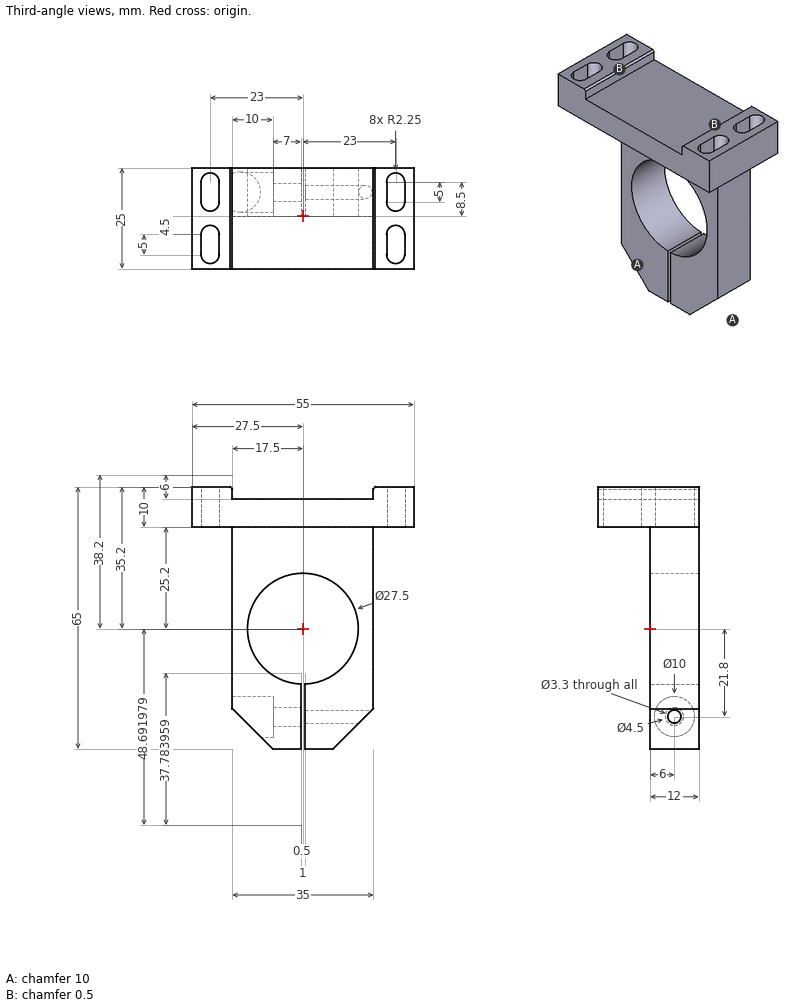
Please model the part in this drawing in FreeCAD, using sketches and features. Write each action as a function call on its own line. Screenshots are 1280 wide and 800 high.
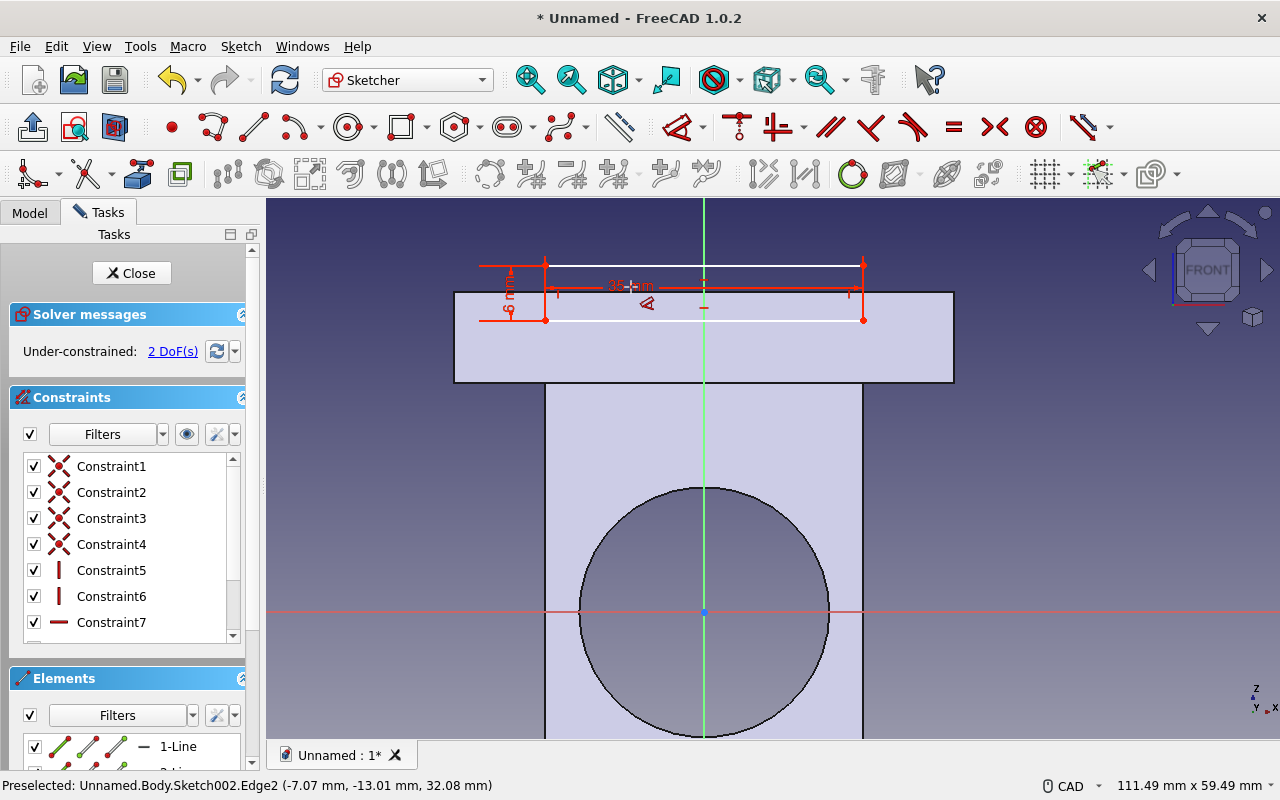
click(545, 266)
click(625, 646)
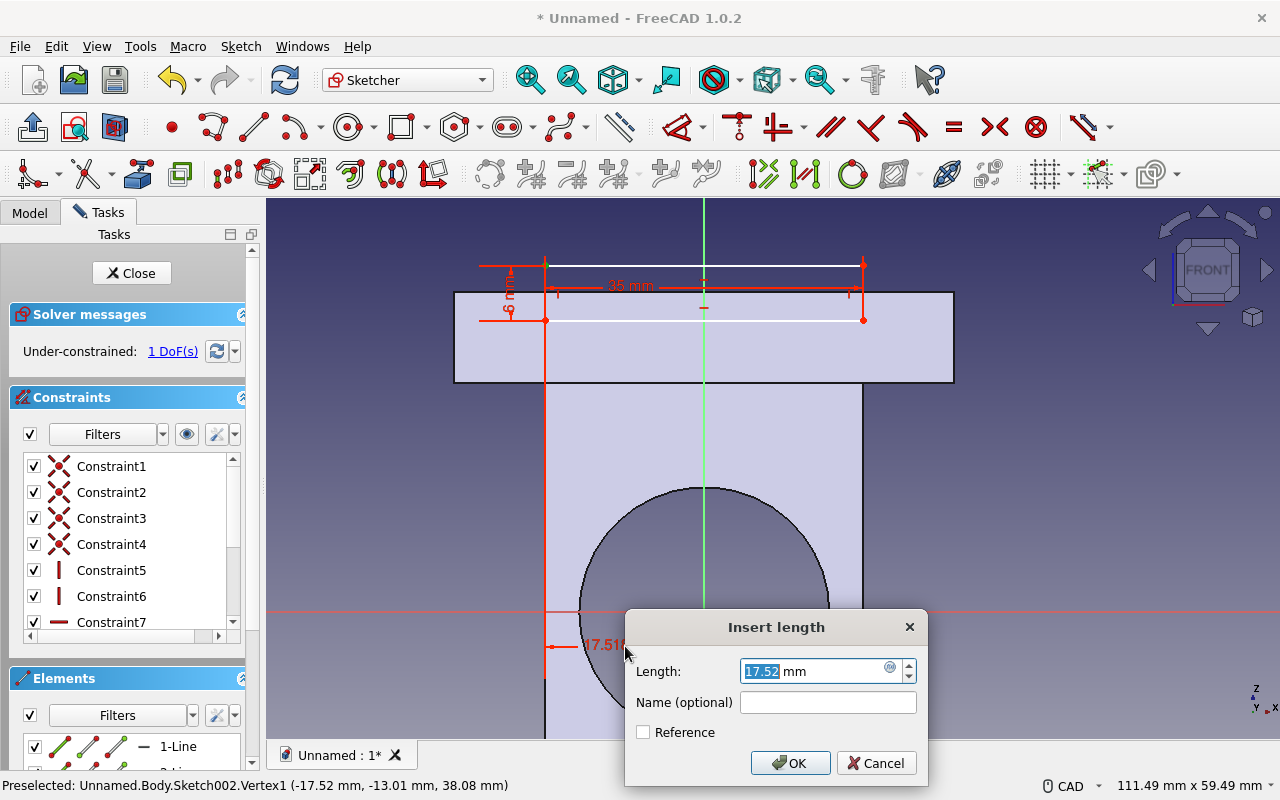
text(17.5)
key(Return)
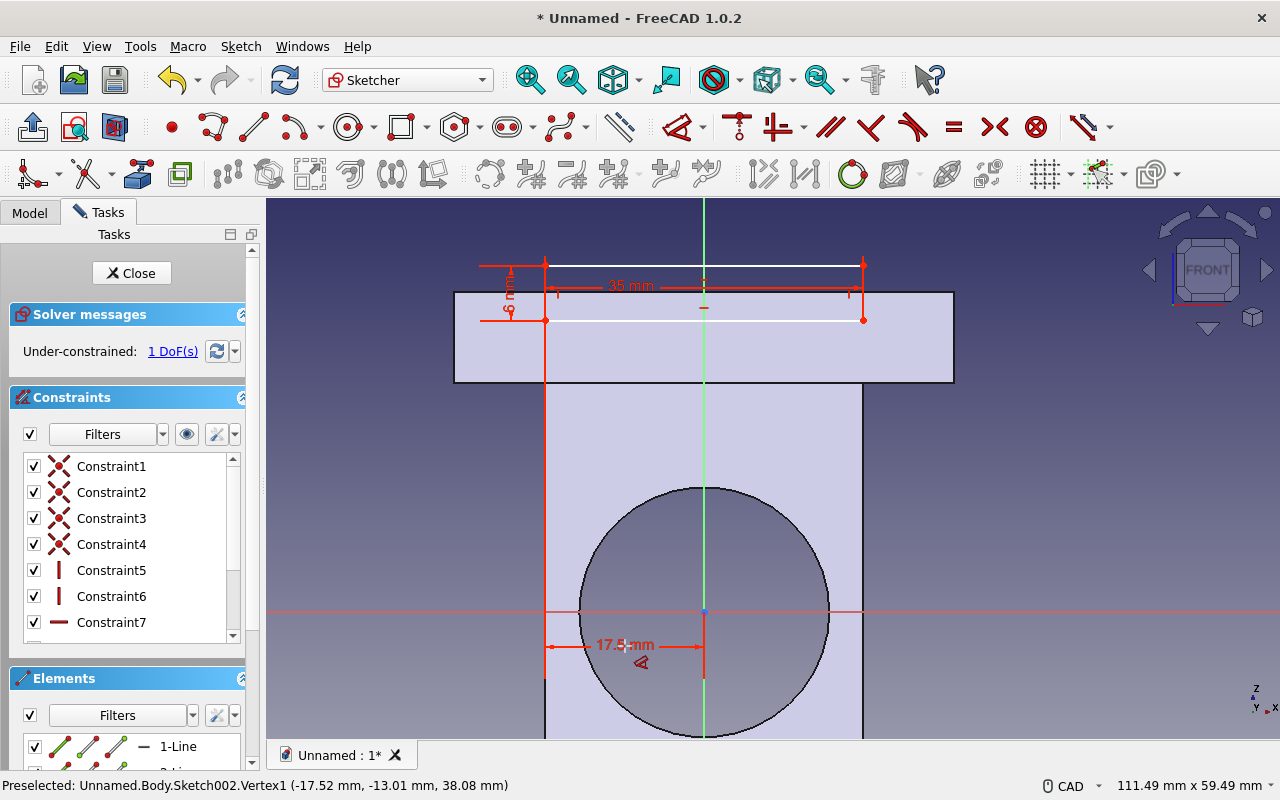
click(545, 266)
click(511, 439)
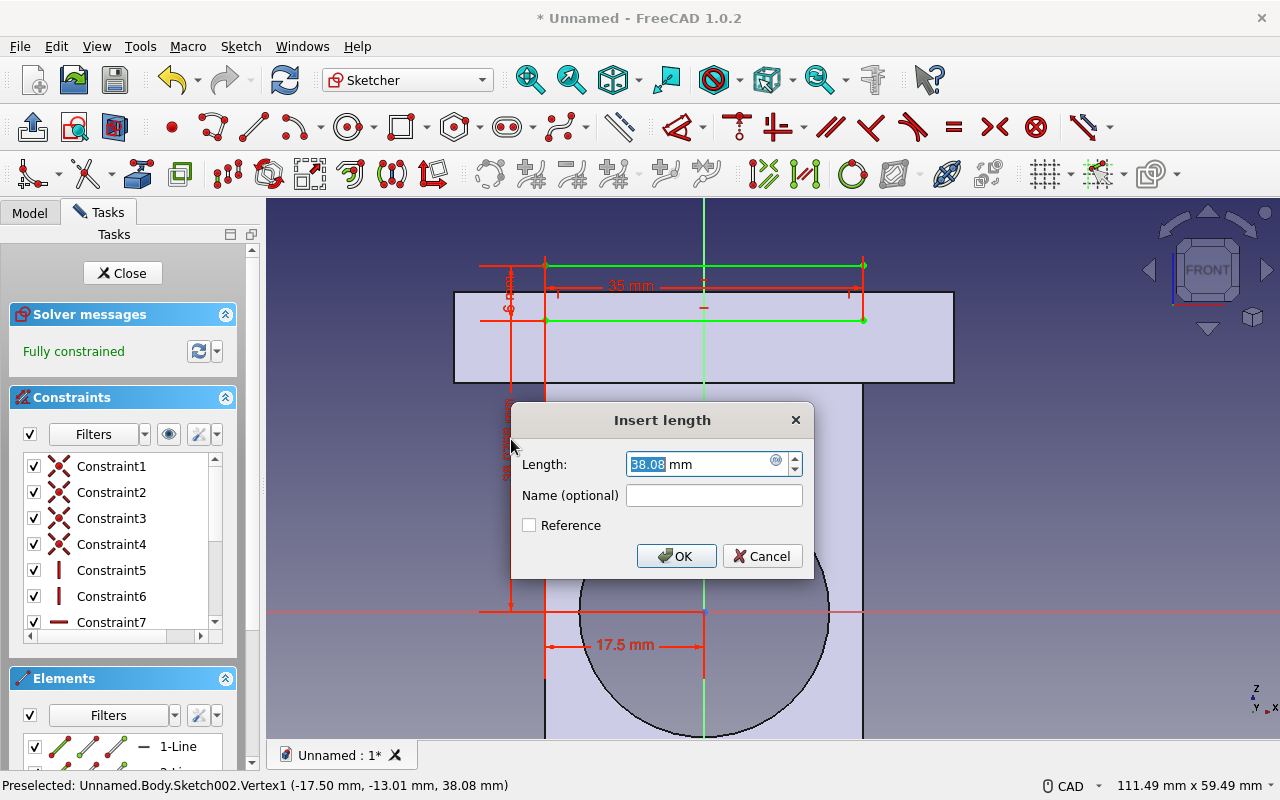
text(38.2)
key(Return)
key(Escape)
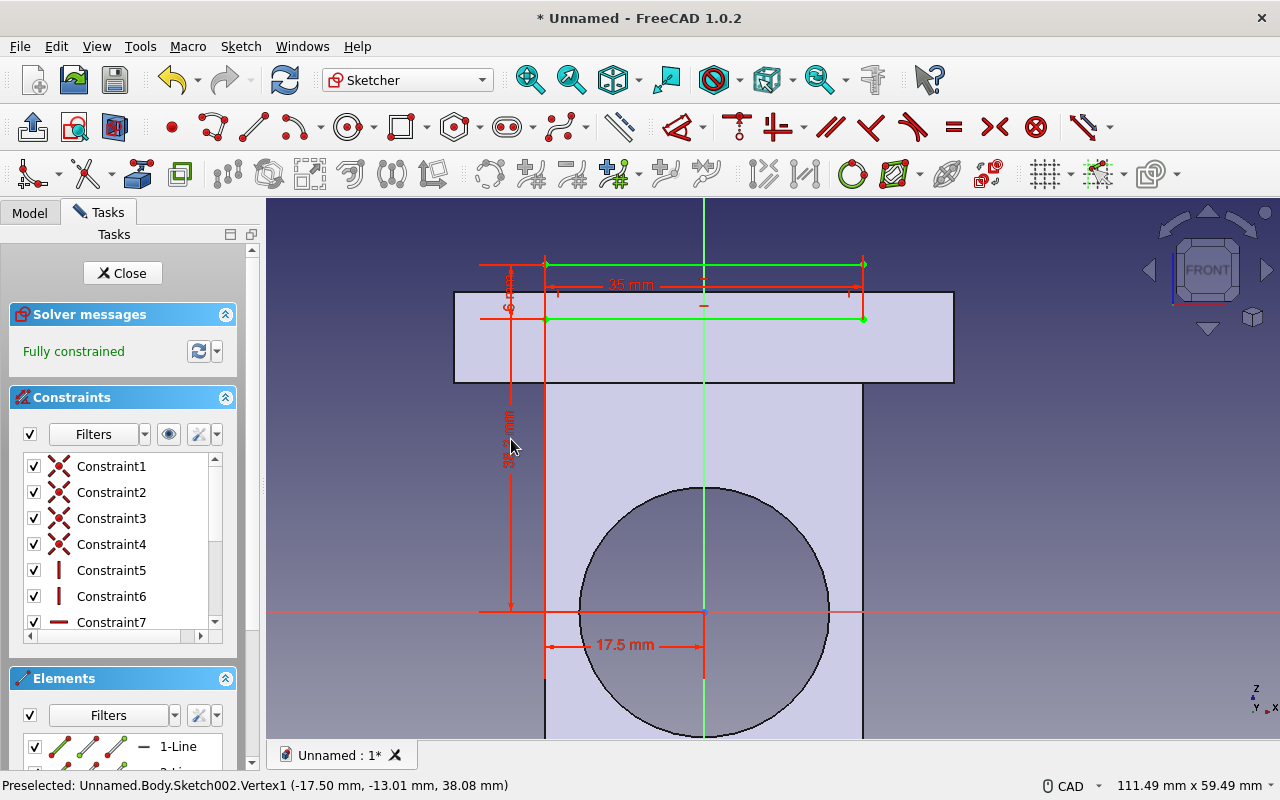
click(123, 273)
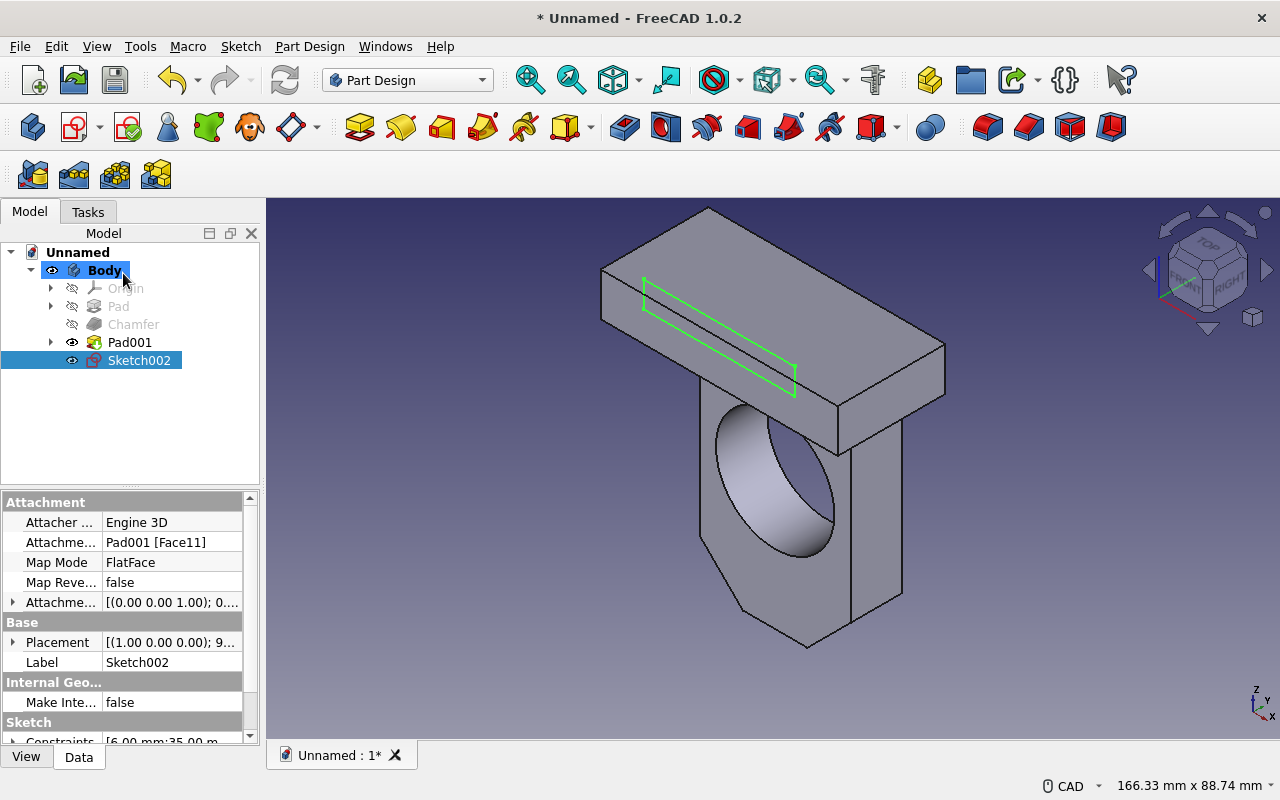
click(625, 128)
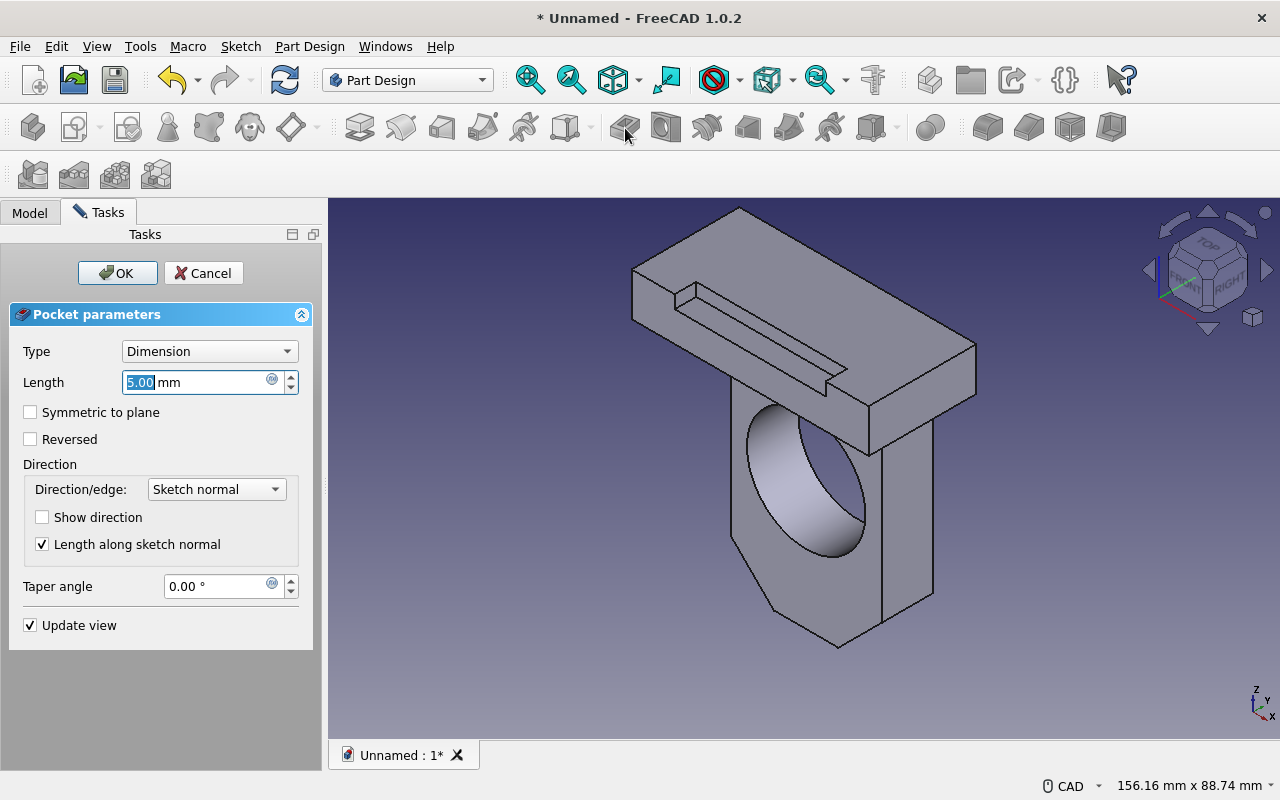
click(210, 352)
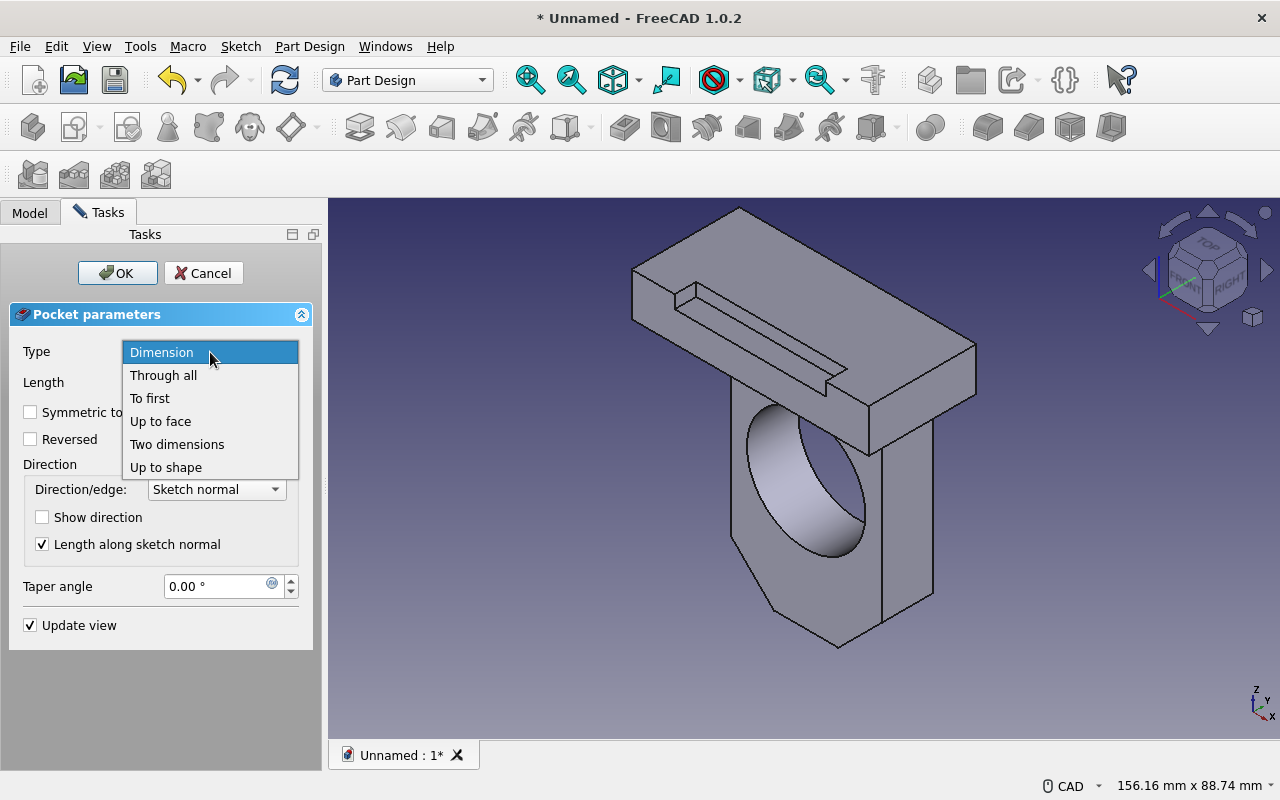
click(208, 376)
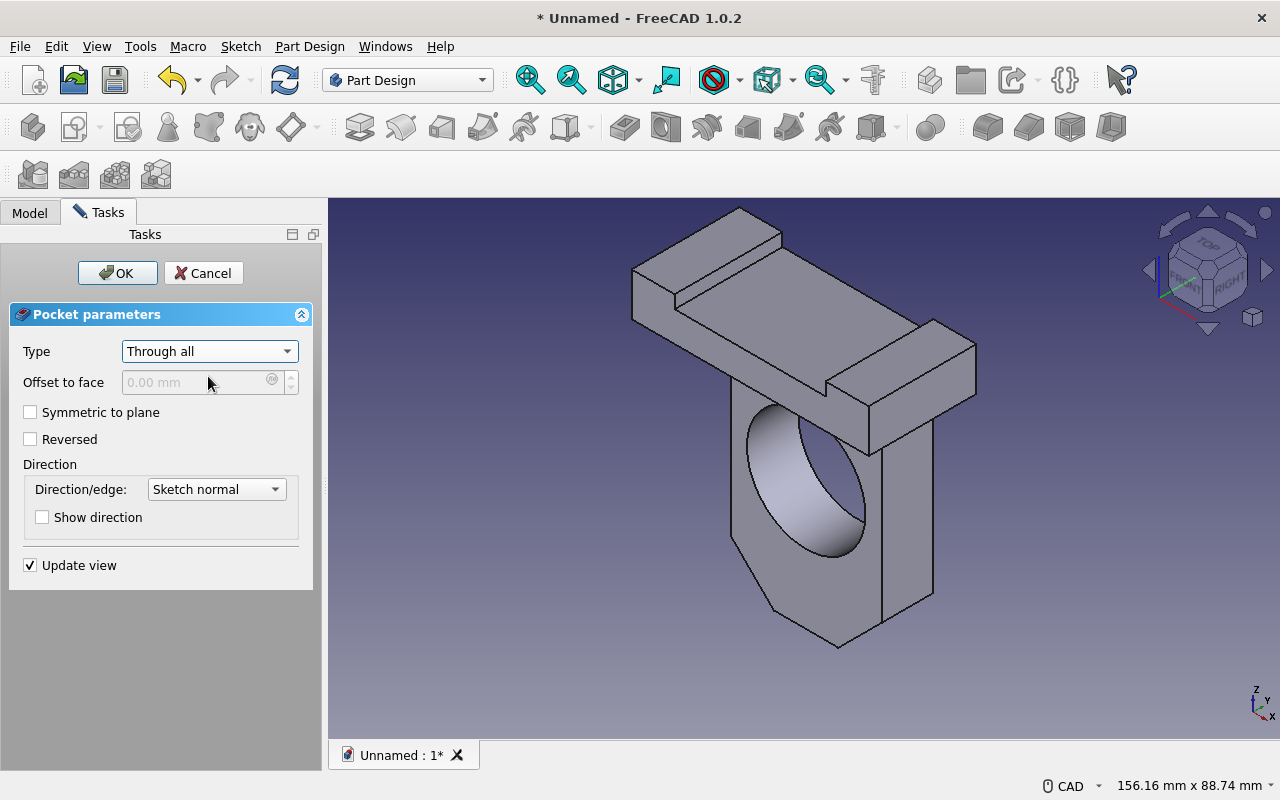
click(118, 273)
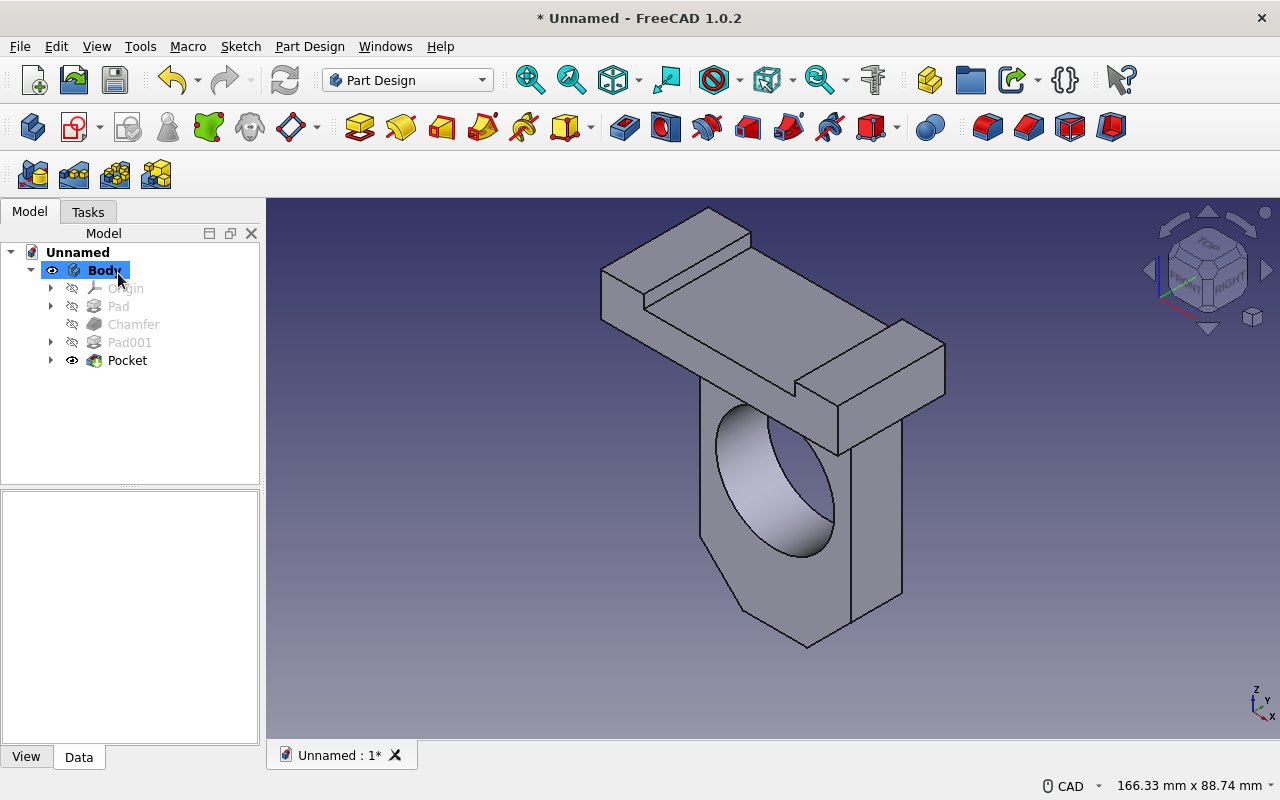
key(5)